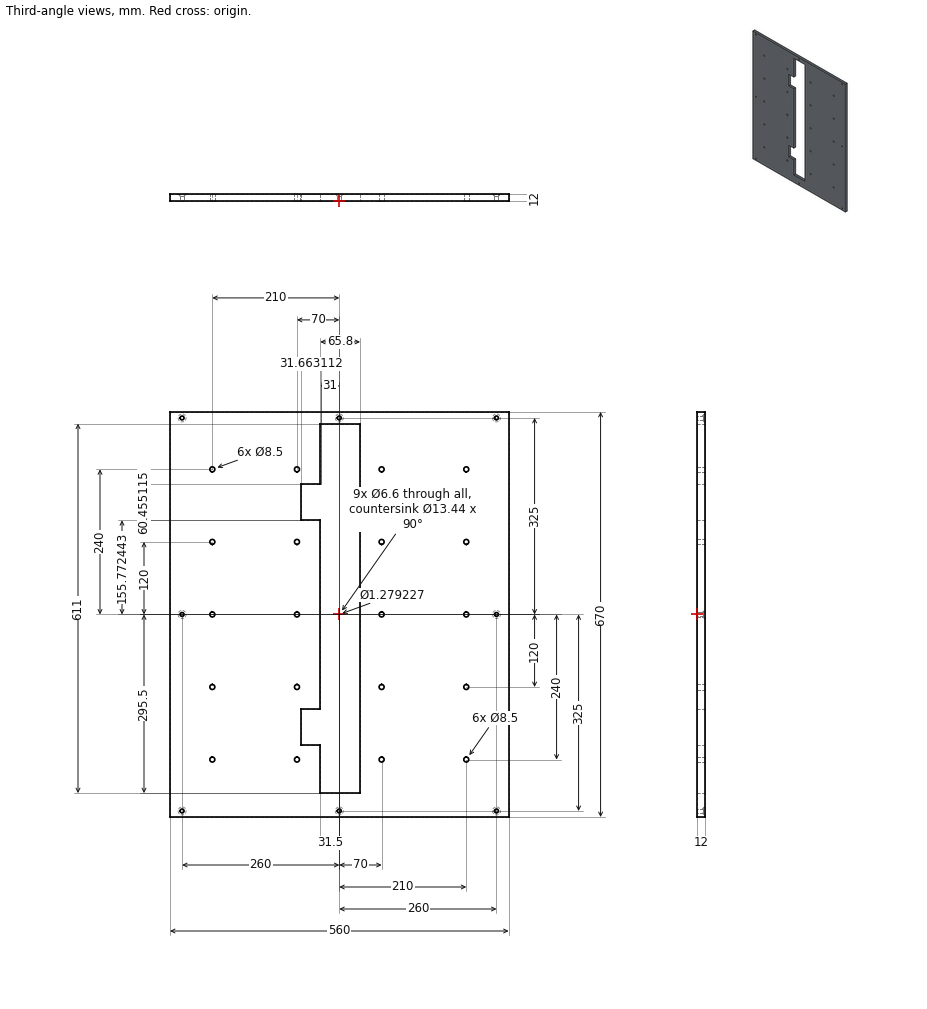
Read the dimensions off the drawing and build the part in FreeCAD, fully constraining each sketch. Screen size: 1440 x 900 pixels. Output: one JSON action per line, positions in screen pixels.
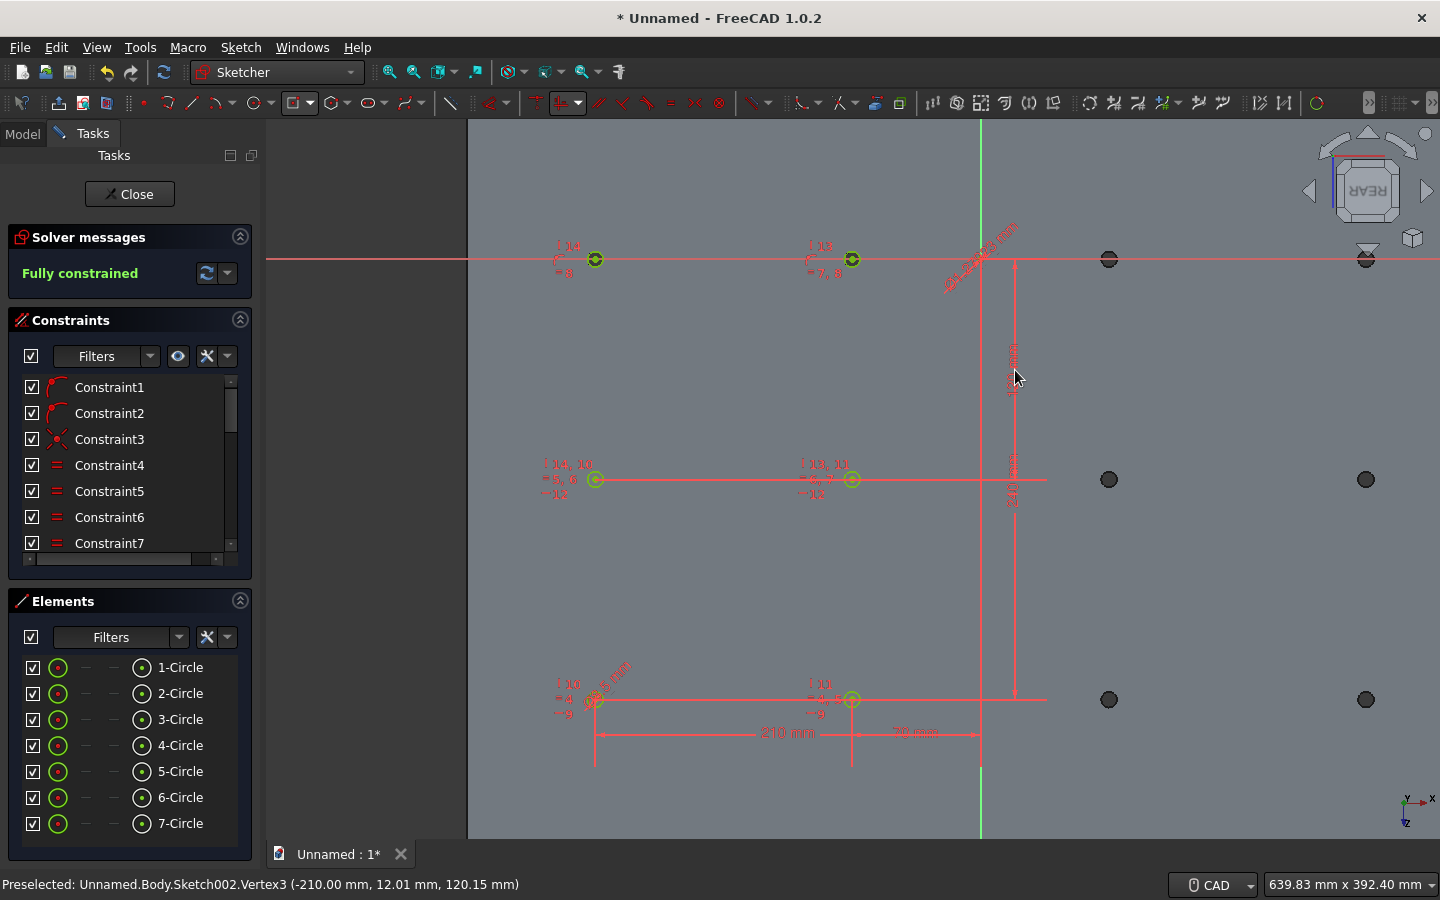
{"action": "left_click", "coordinate": [130, 194]}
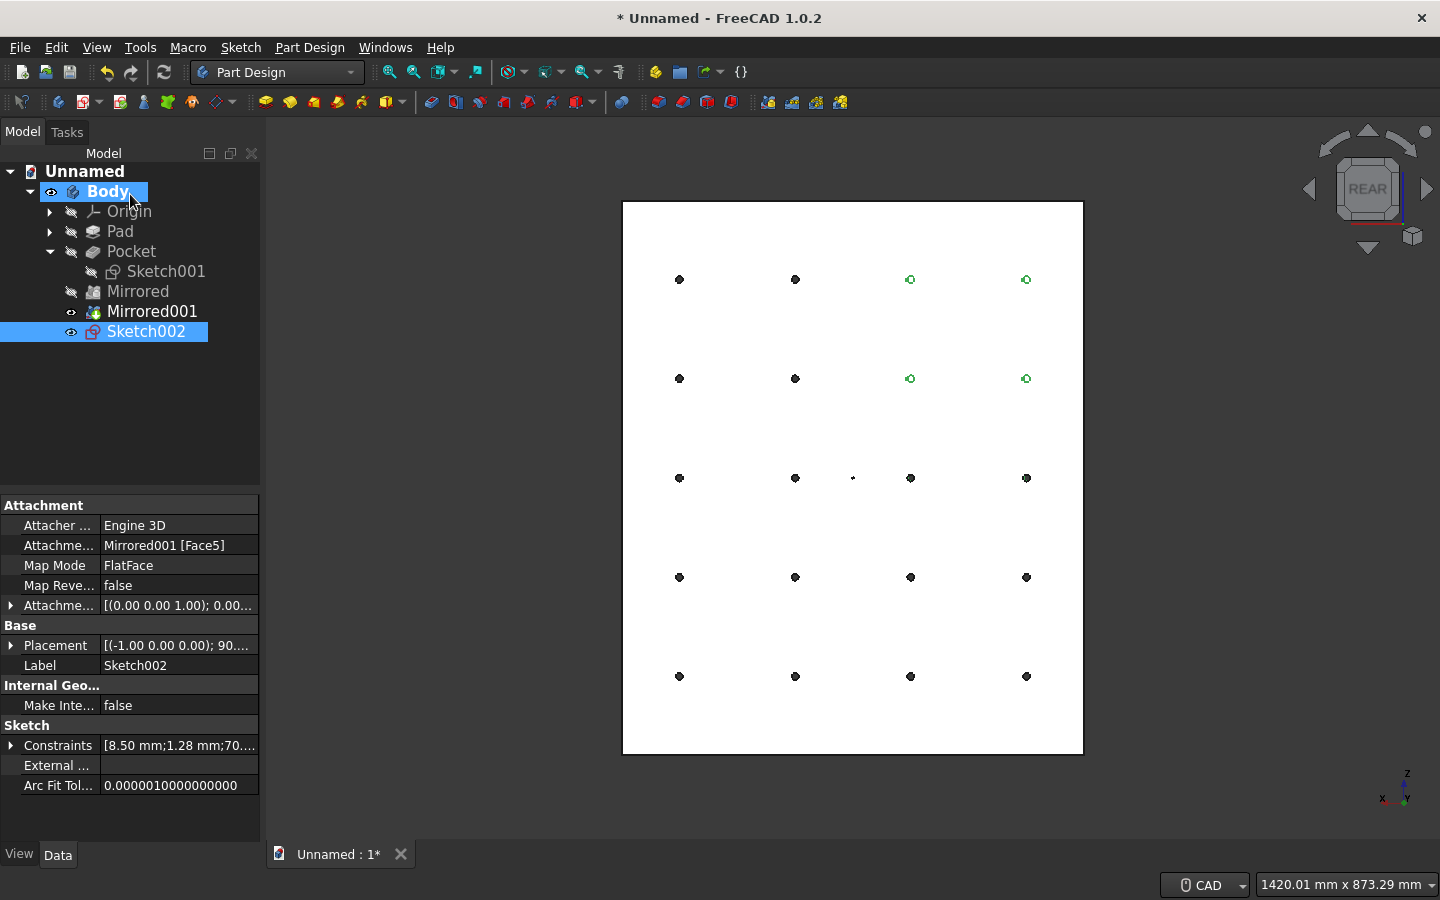
{"action": "left_click", "coordinate": [432, 102]}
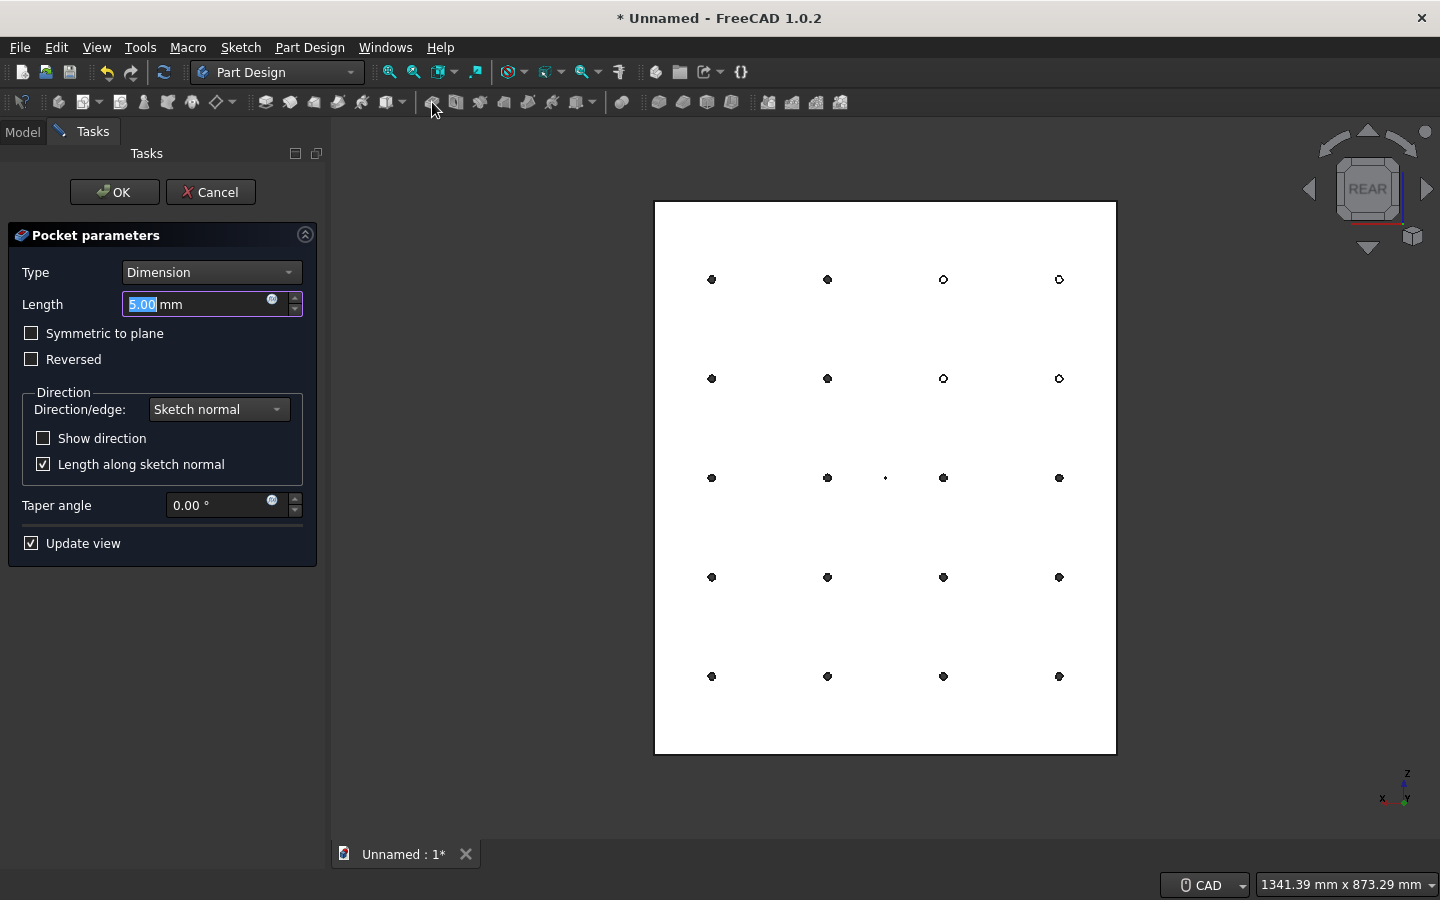
{"action": "type", "text": "12"}
{"action": "key", "text": "Tab"}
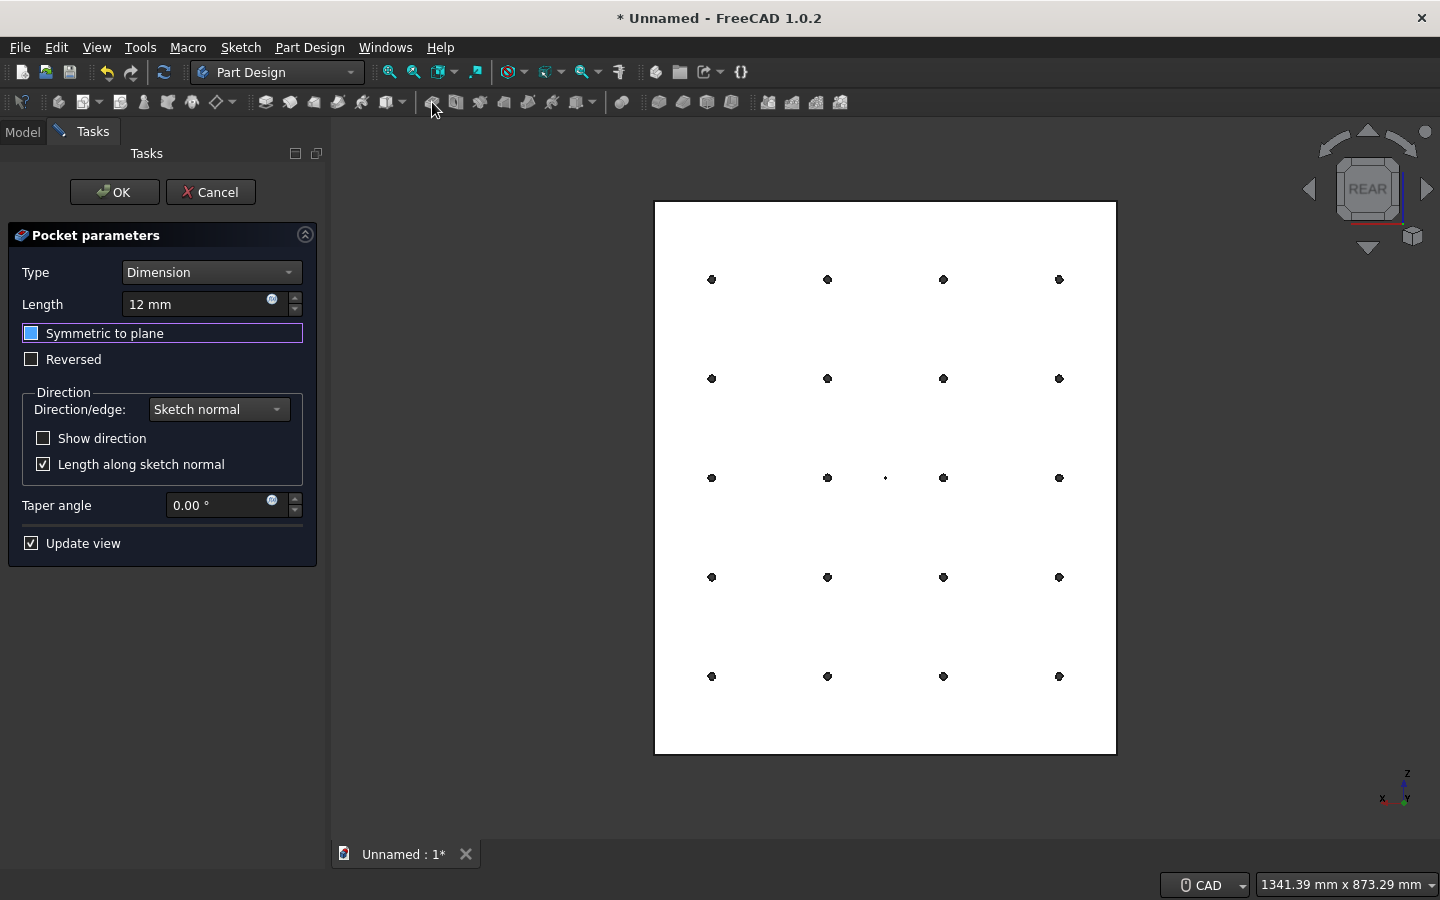
{"action": "left_click", "coordinate": [115, 192]}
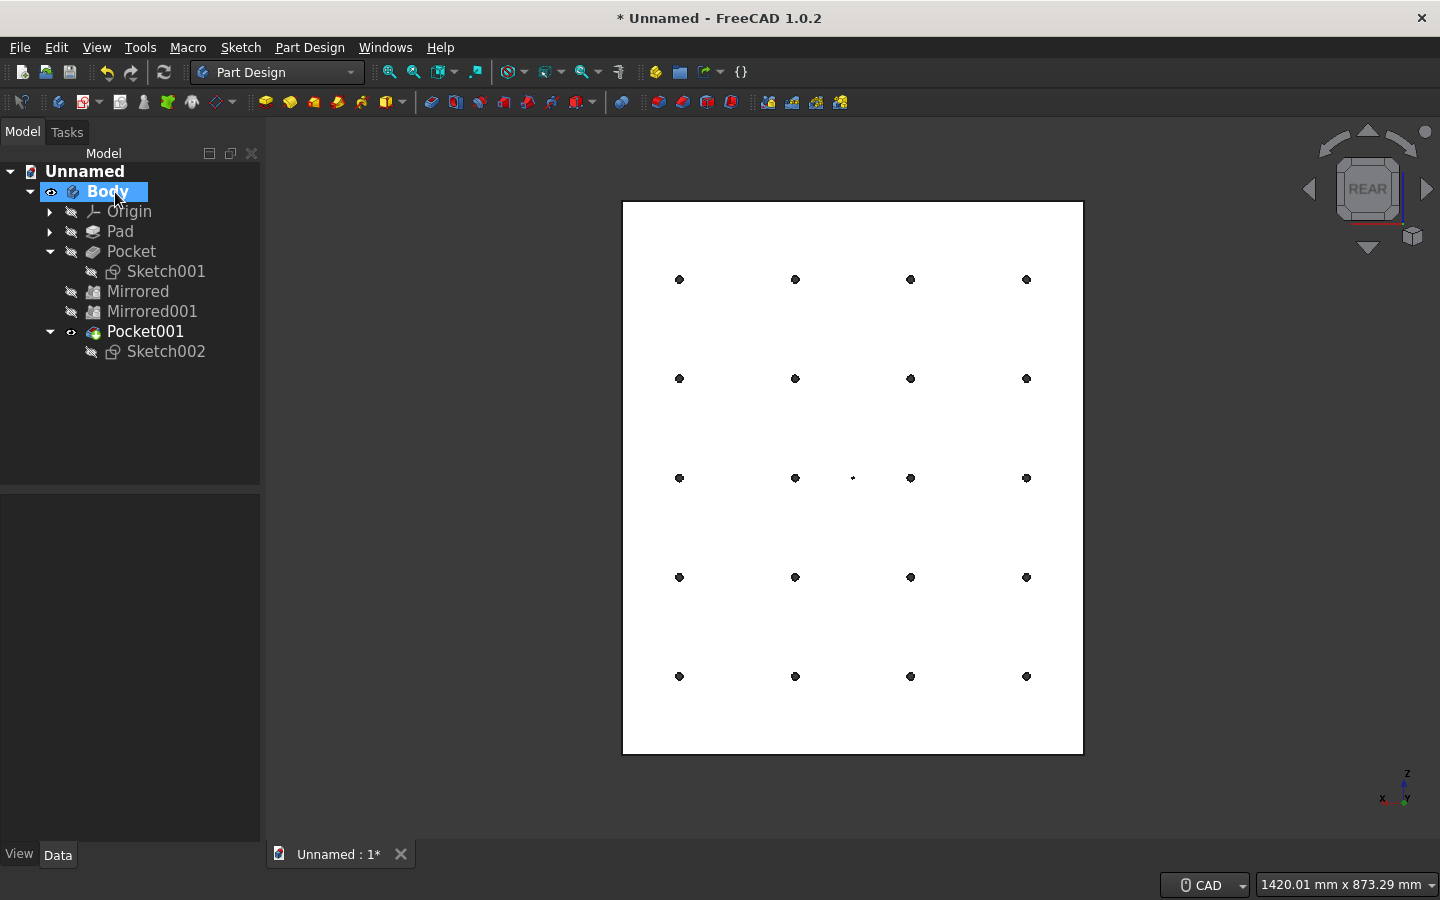
{"action": "left_click", "coordinate": [853, 635]}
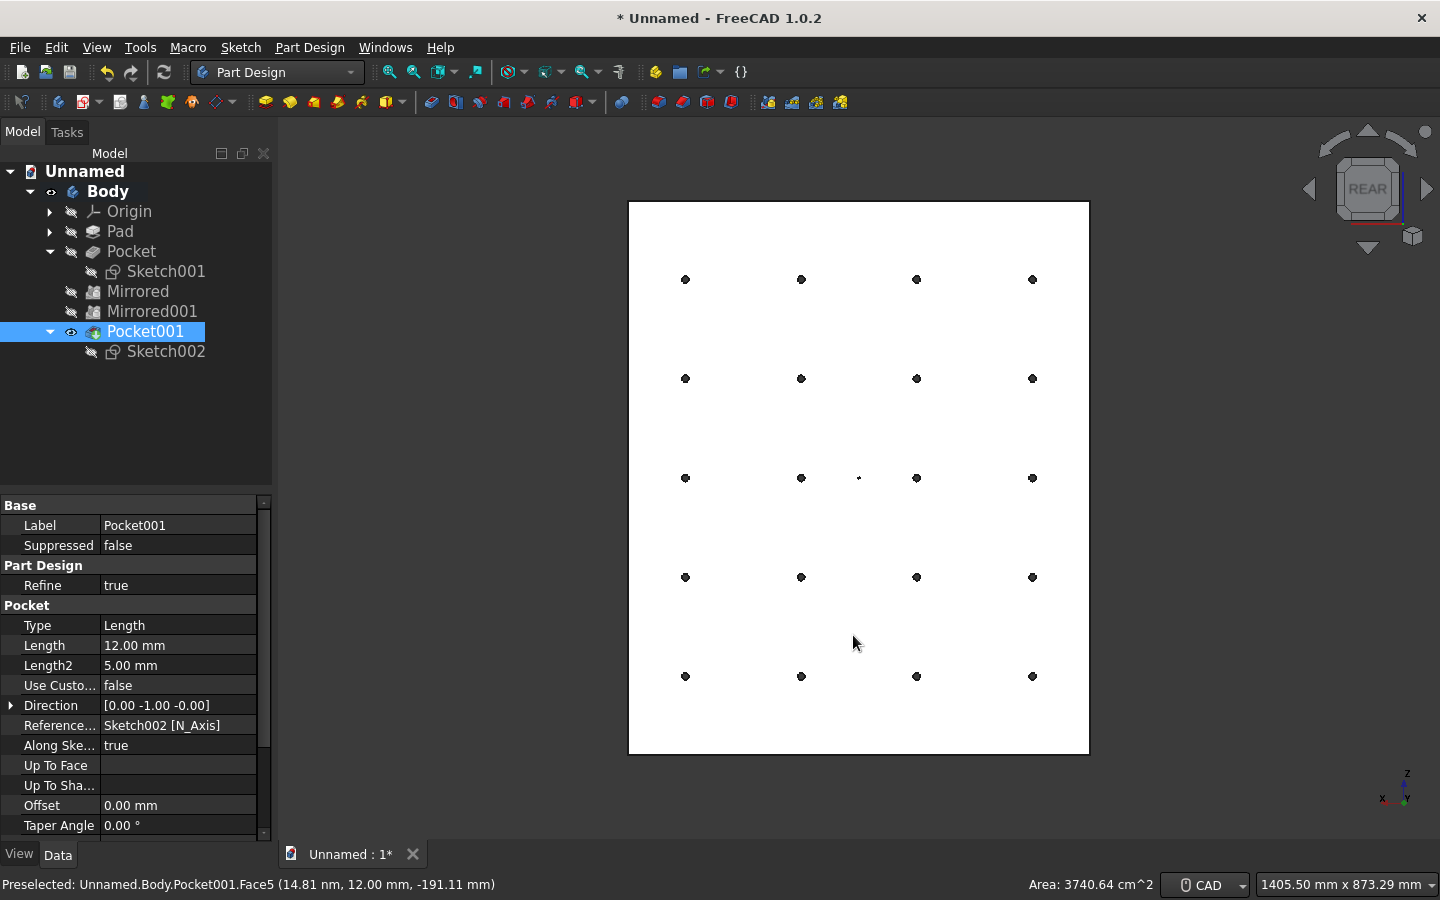
{"action": "left_click", "coordinate": [84, 102]}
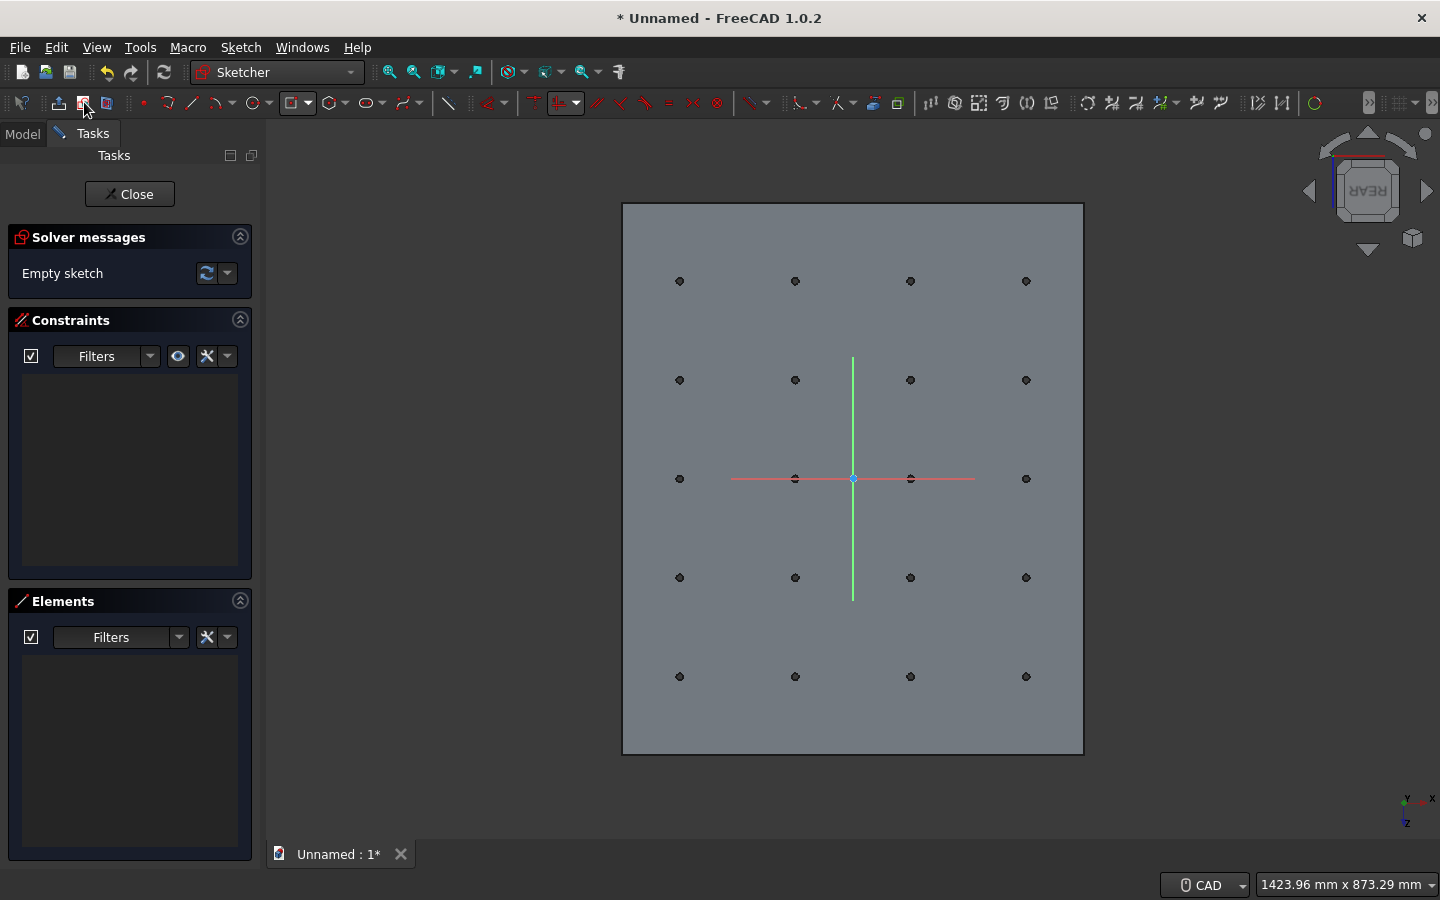
{"action": "left_click", "coordinate": [254, 104]}